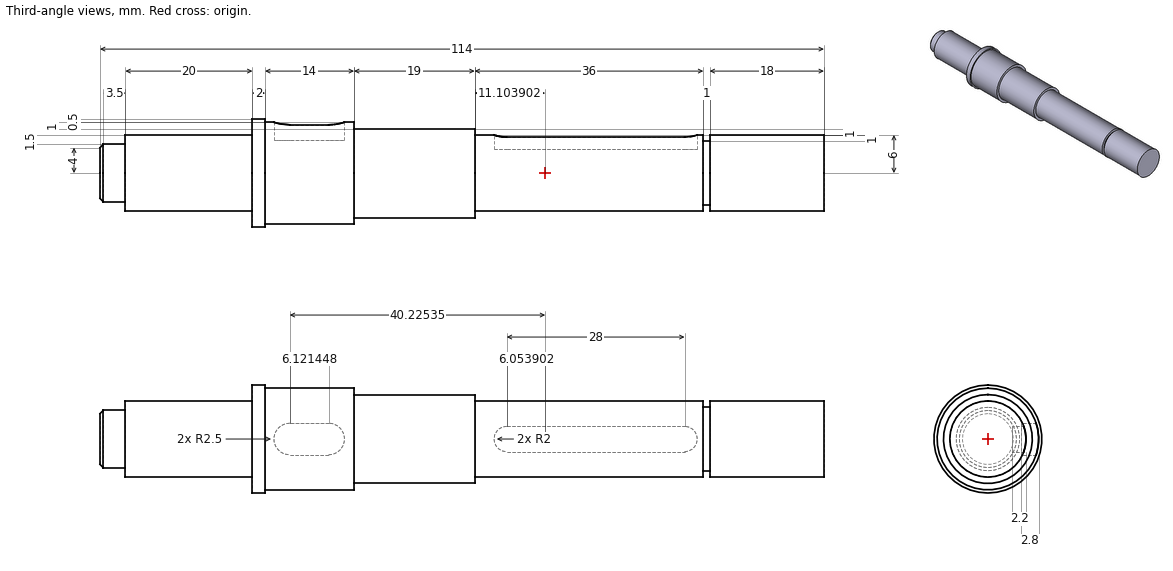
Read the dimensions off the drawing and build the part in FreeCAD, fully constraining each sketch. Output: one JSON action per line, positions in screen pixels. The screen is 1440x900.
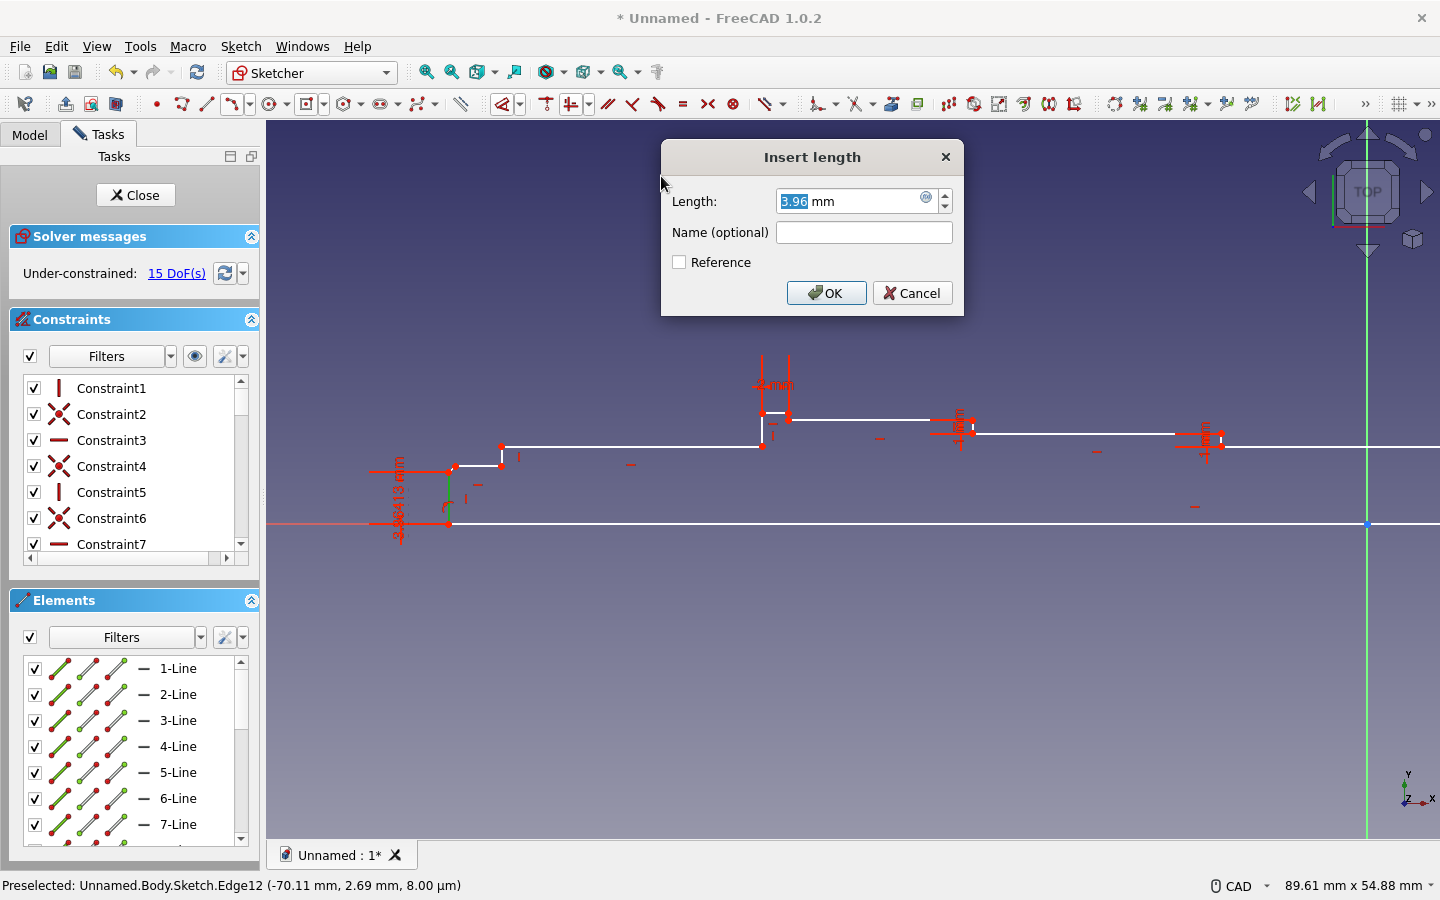
{"action": "type", "text": "4"}
{"action": "key", "text": "Return"}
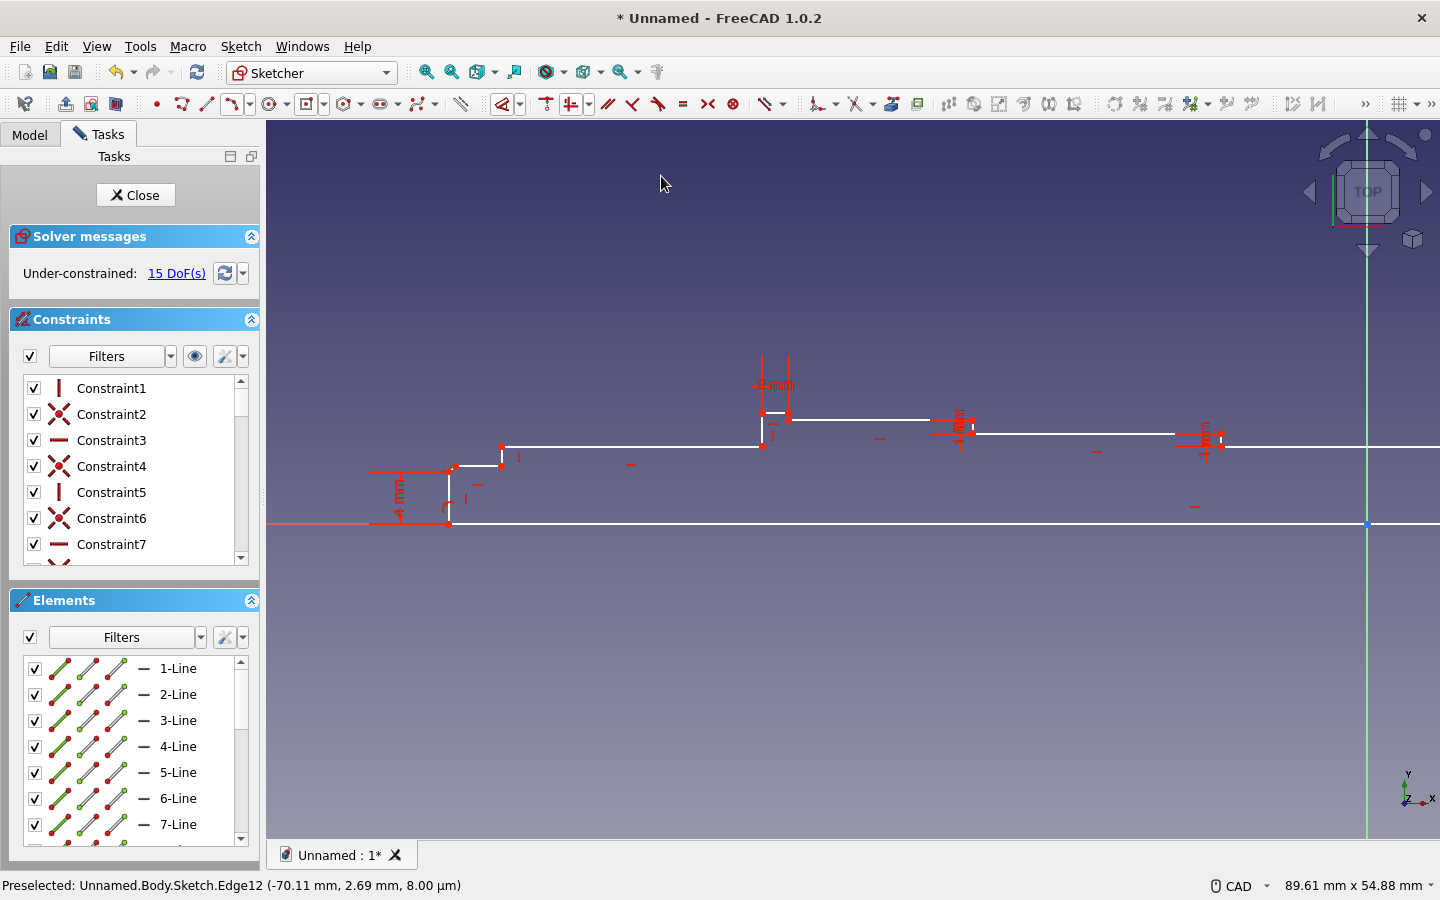
{"action": "scroll", "coordinate": [449, 488], "scroll_direction": "down", "scroll_amount": 4}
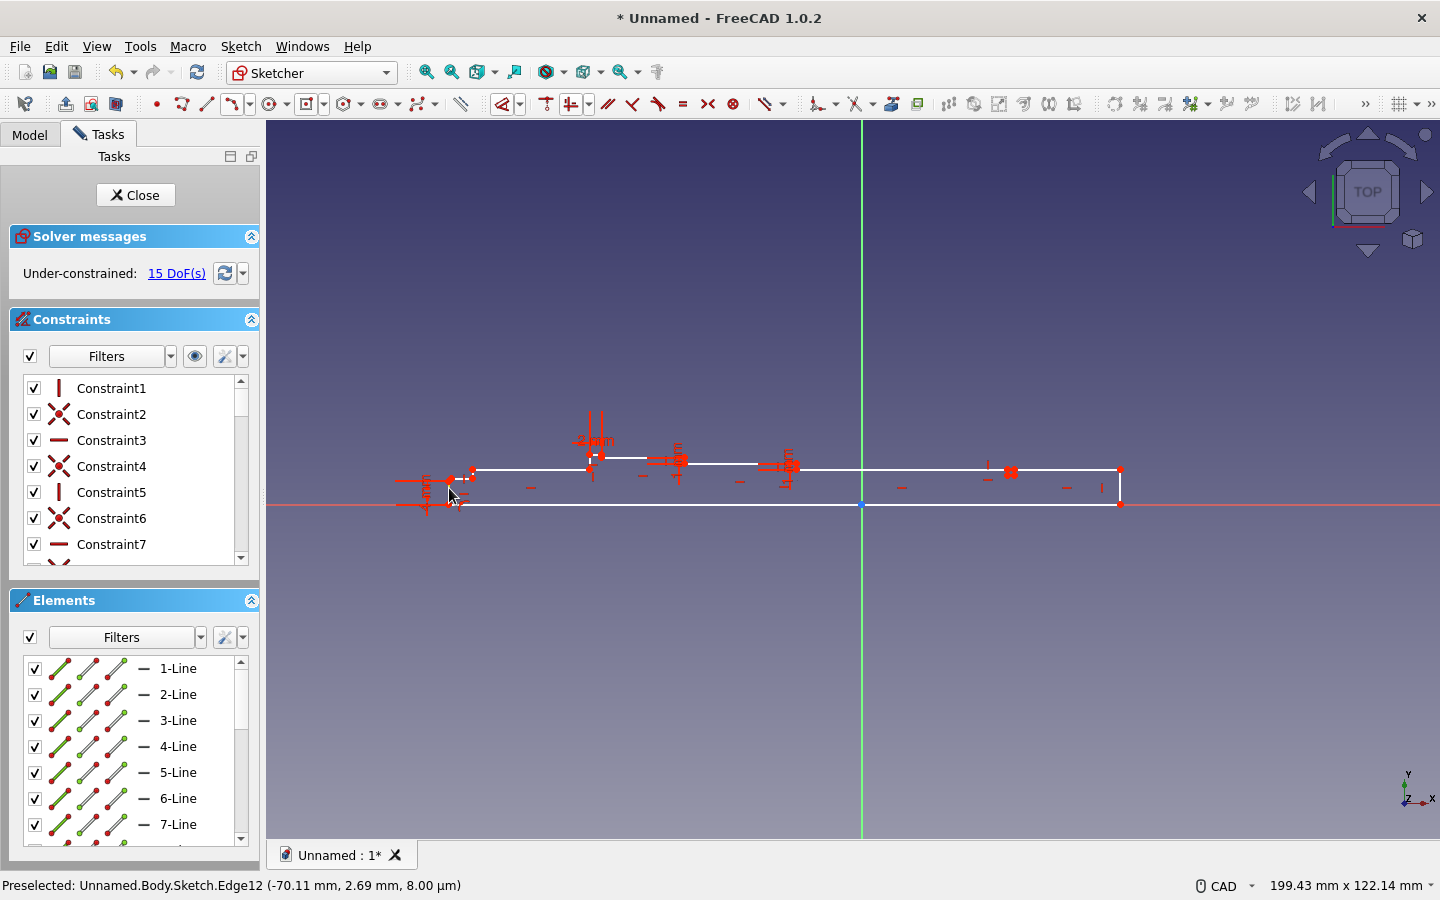
{"action": "scroll", "coordinate": [1120, 494], "scroll_direction": "up", "scroll_amount": 2}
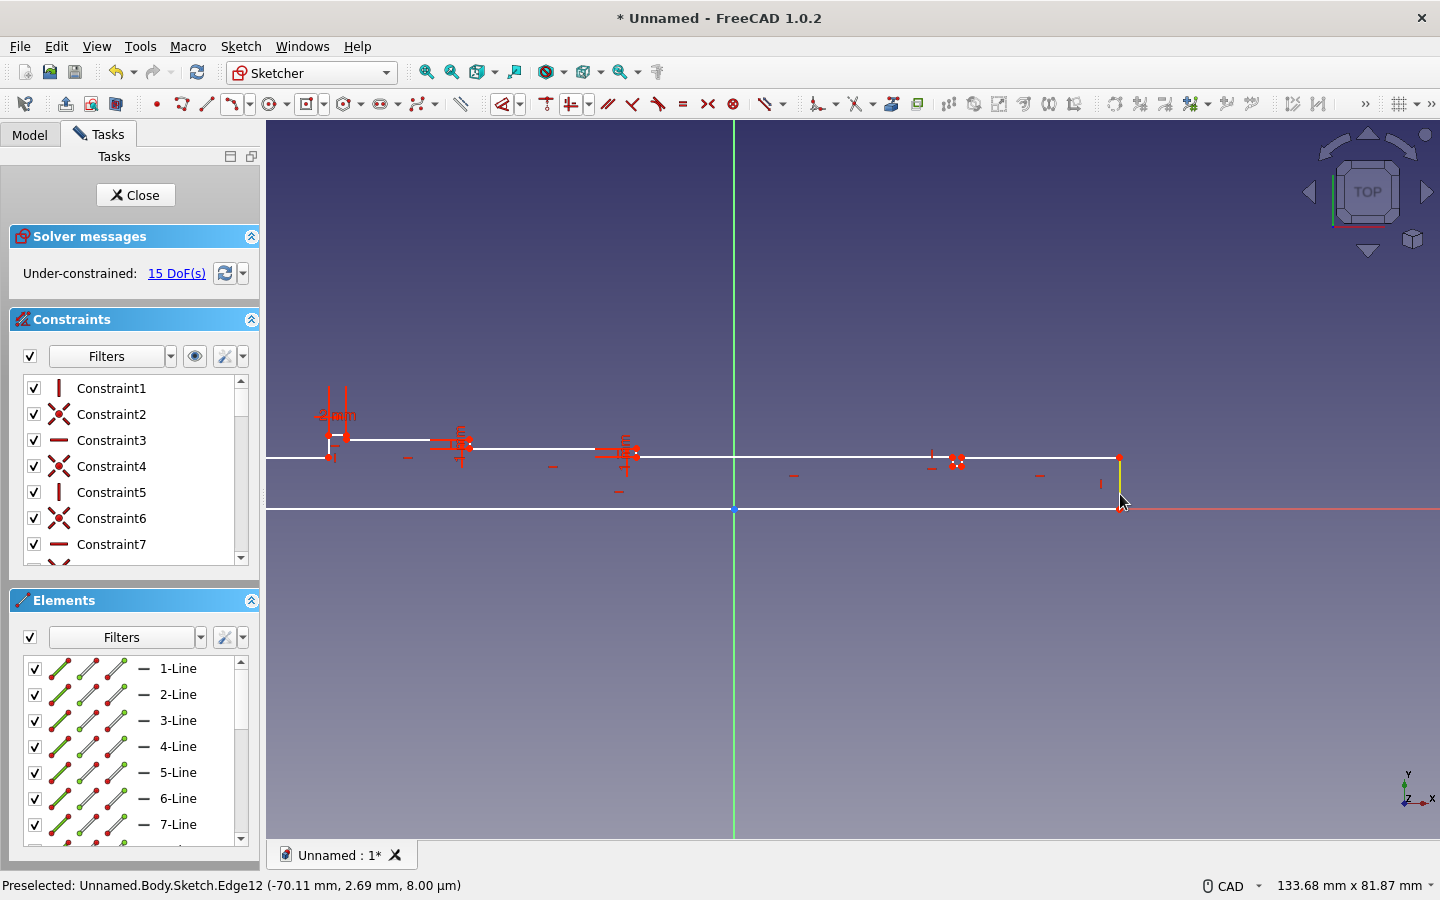
{"action": "left_click", "coordinate": [1120, 494]}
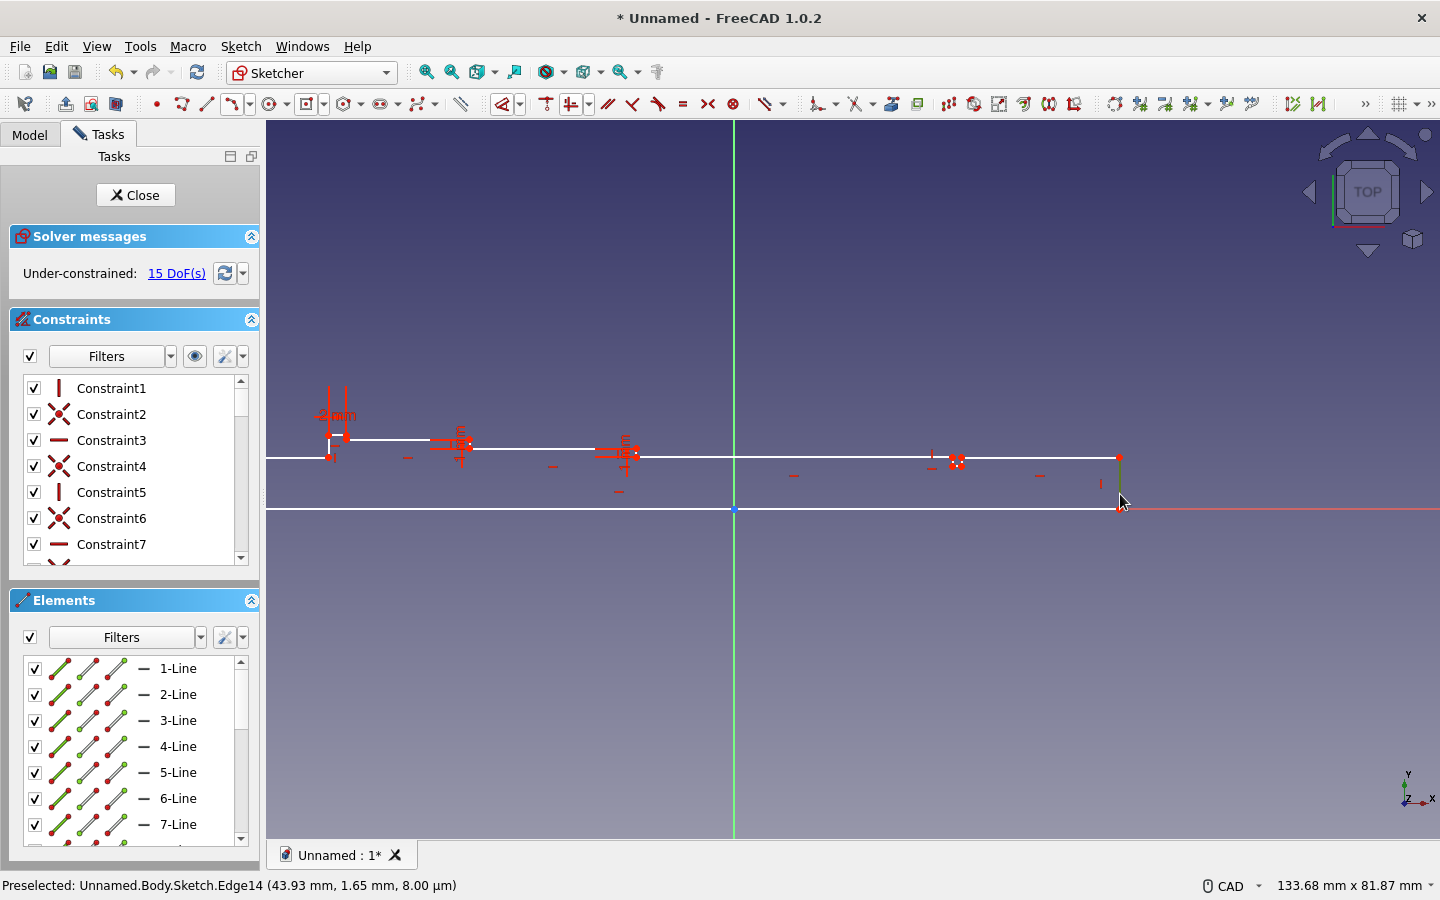
{"action": "key", "text": "i"}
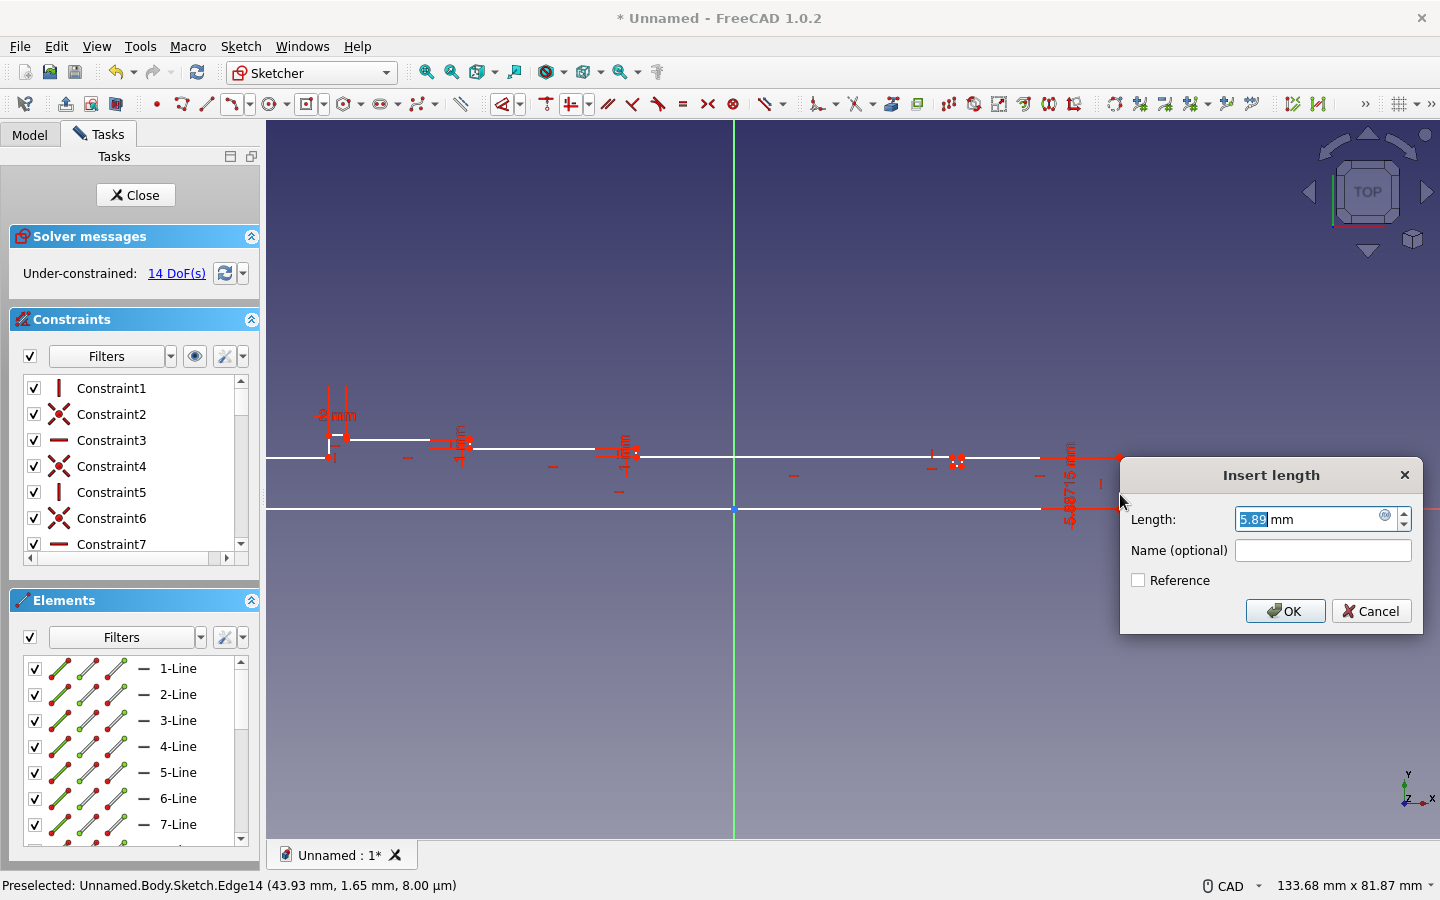
{"action": "type", "text": "6"}
{"action": "key", "text": "Return"}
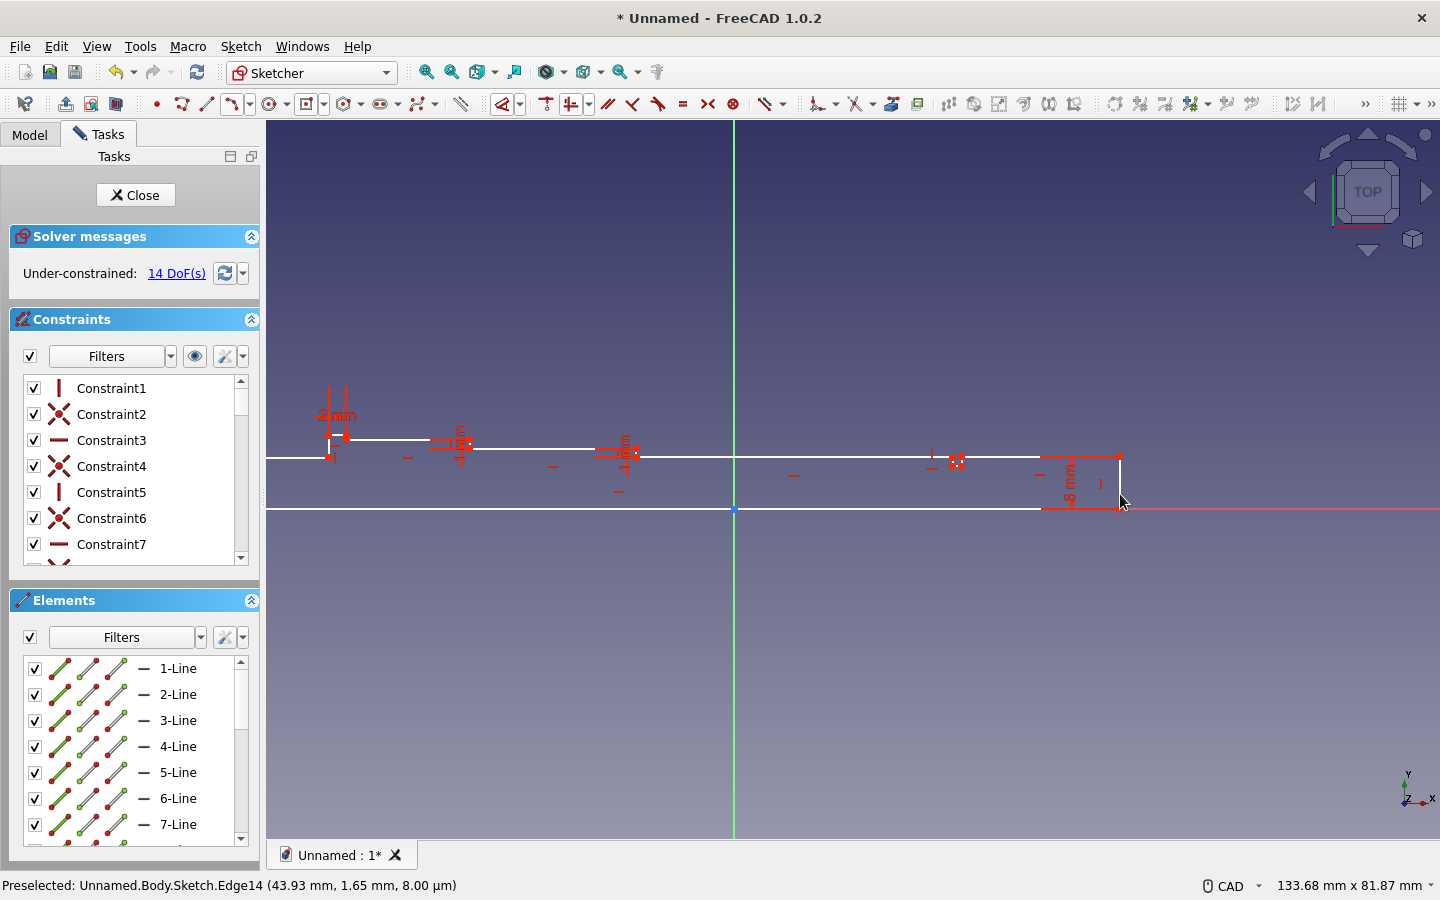
{"action": "scroll", "coordinate": [962, 462], "scroll_direction": "up", "scroll_amount": 8}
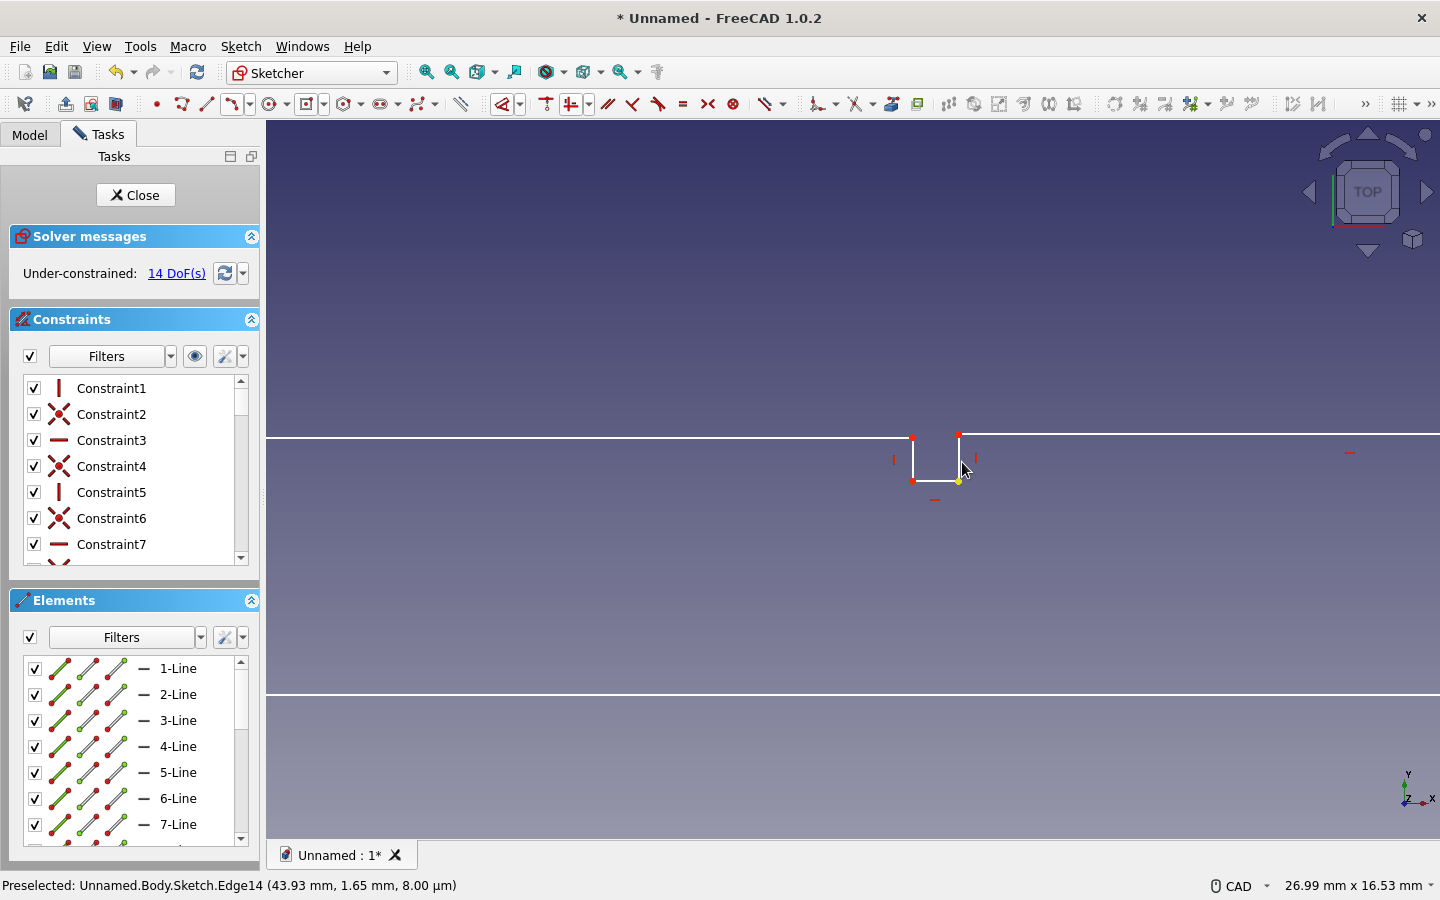
{"action": "left_click", "coordinate": [959, 458]}